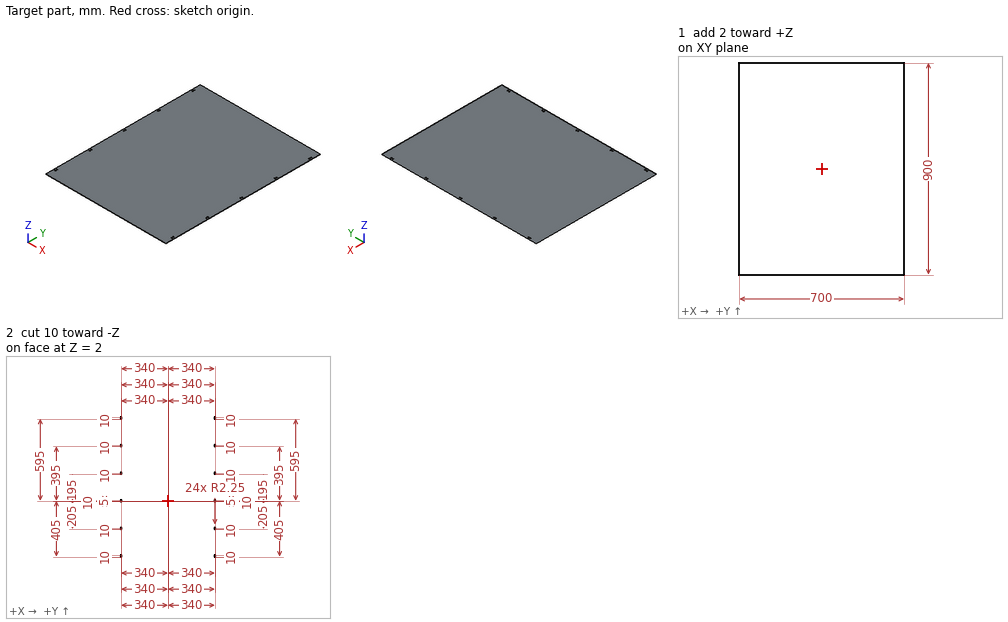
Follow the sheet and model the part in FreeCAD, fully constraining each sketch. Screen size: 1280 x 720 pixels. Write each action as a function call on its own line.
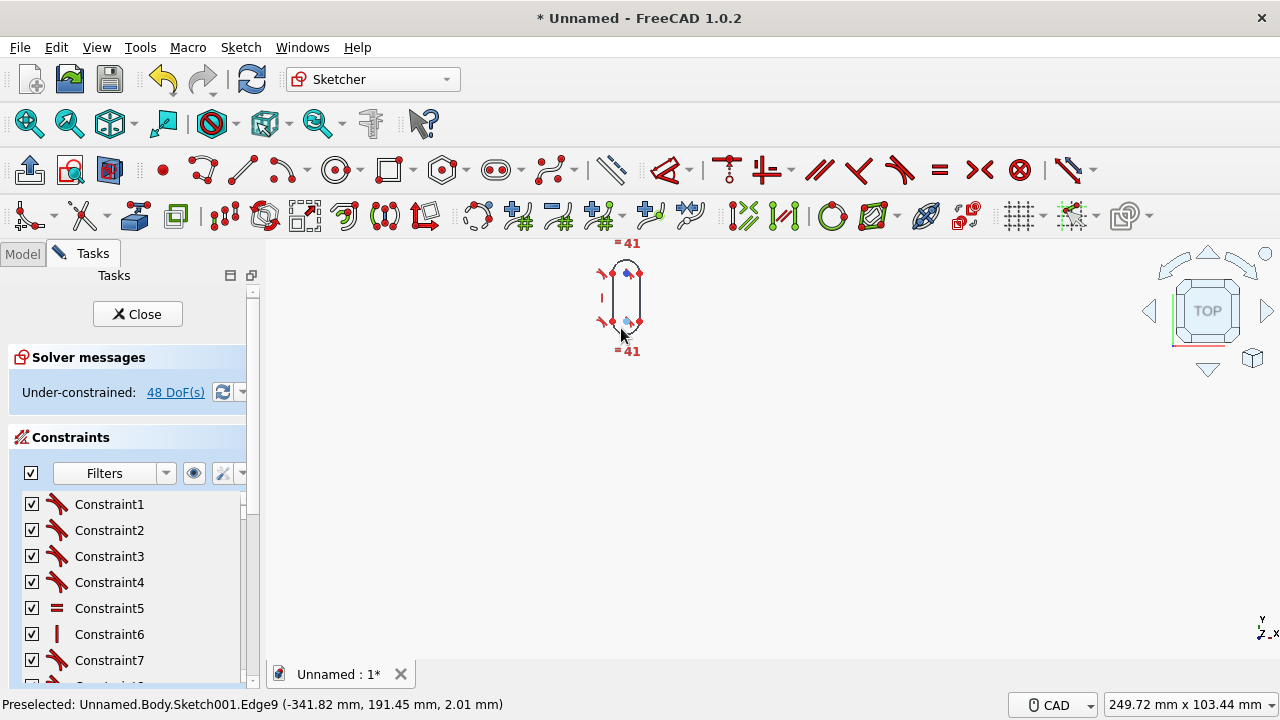
click(618, 332)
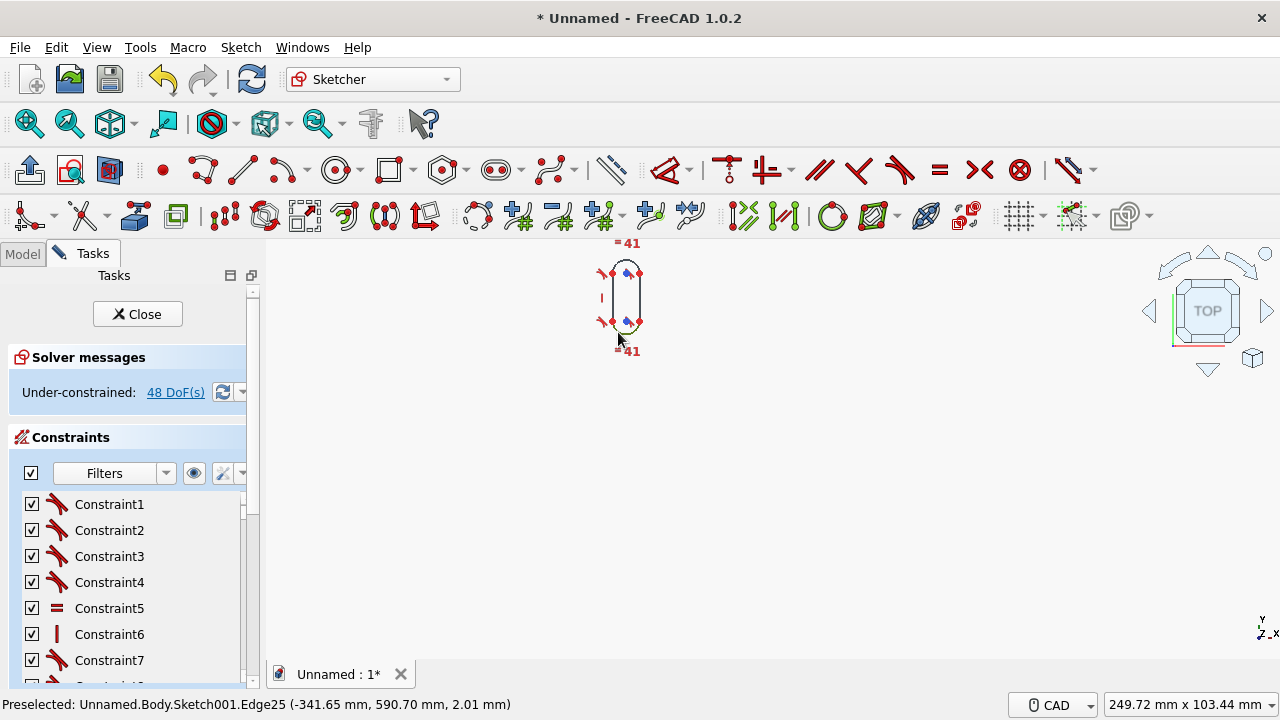
scroll(620, 328, down, 14)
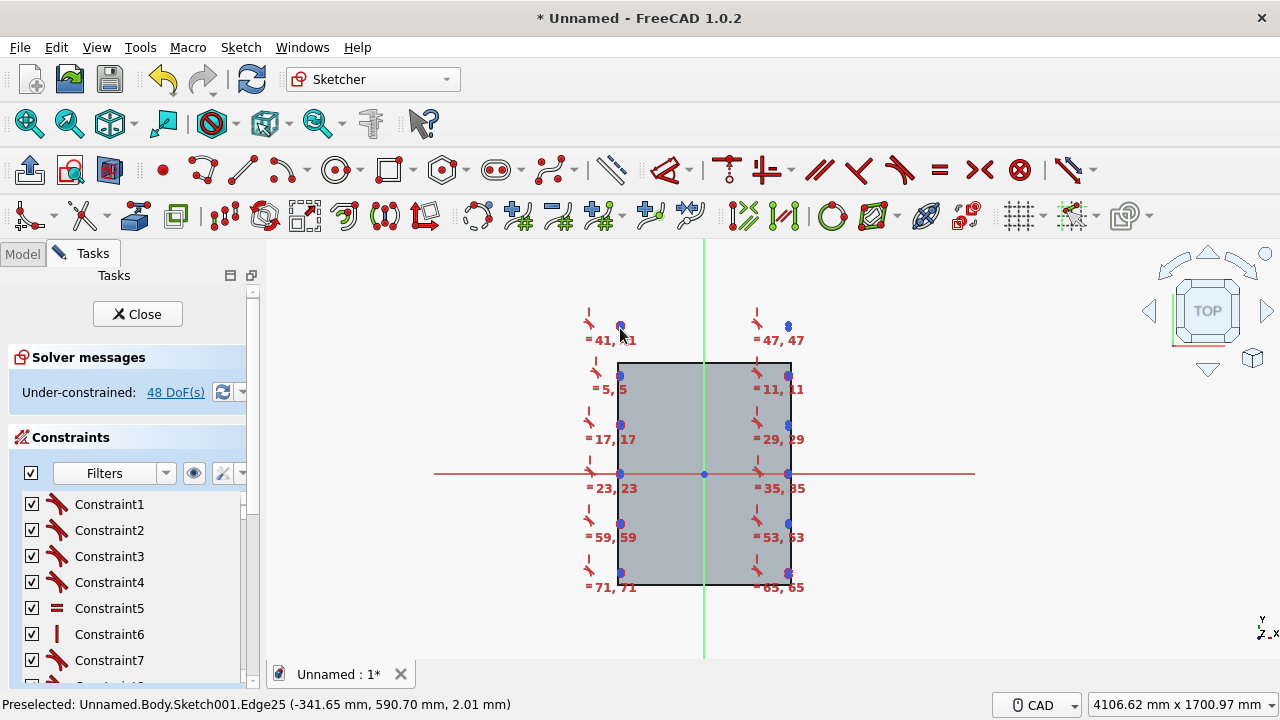
scroll(789, 328, up, 14)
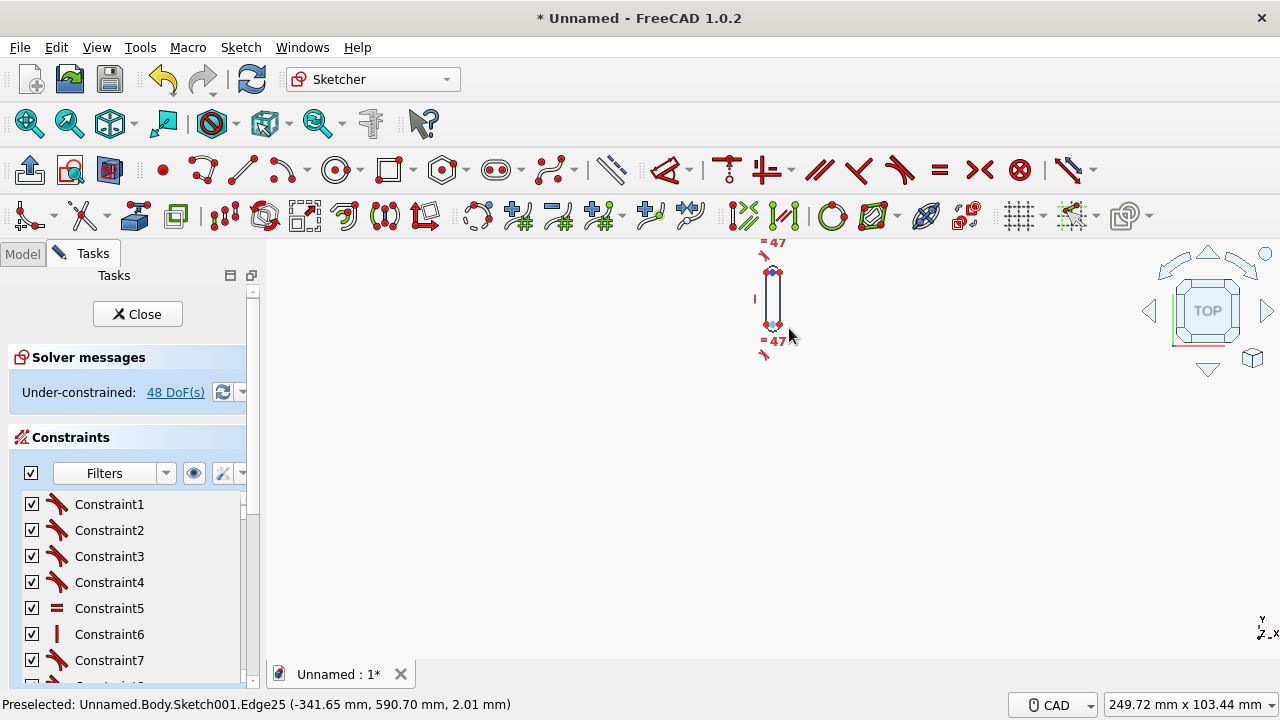
click(773, 332)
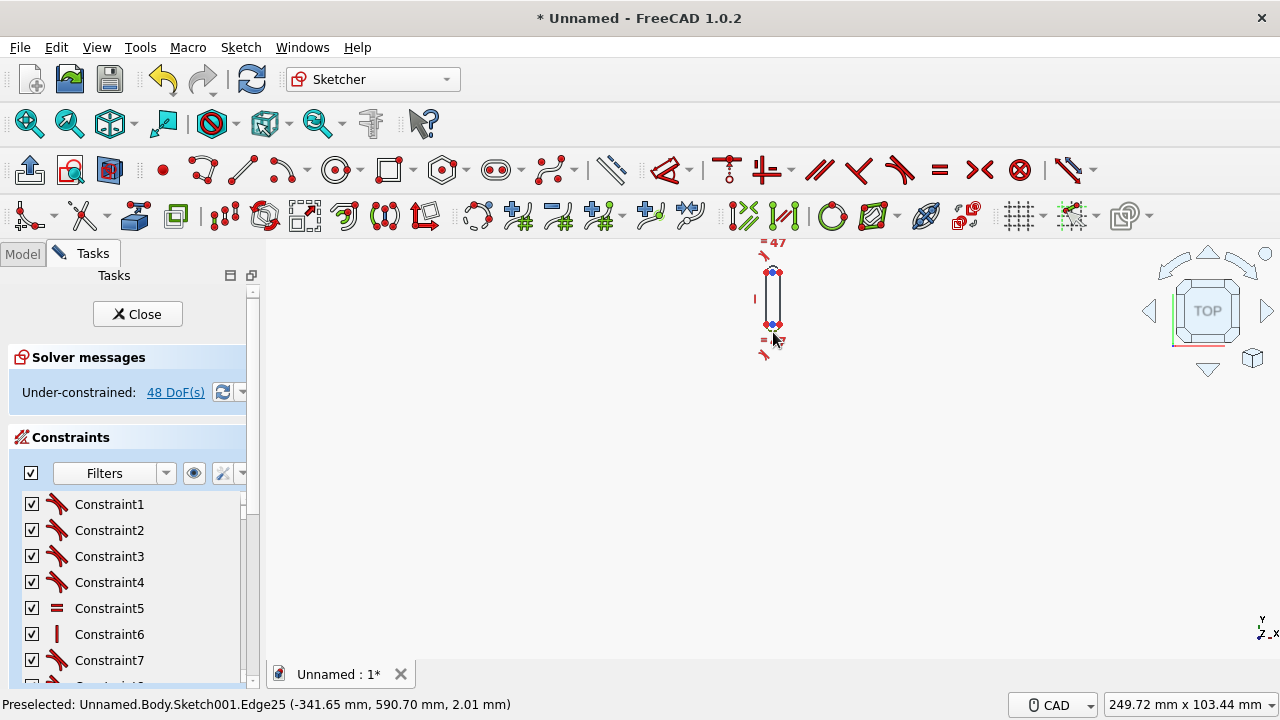
scroll(790, 328, down, 14)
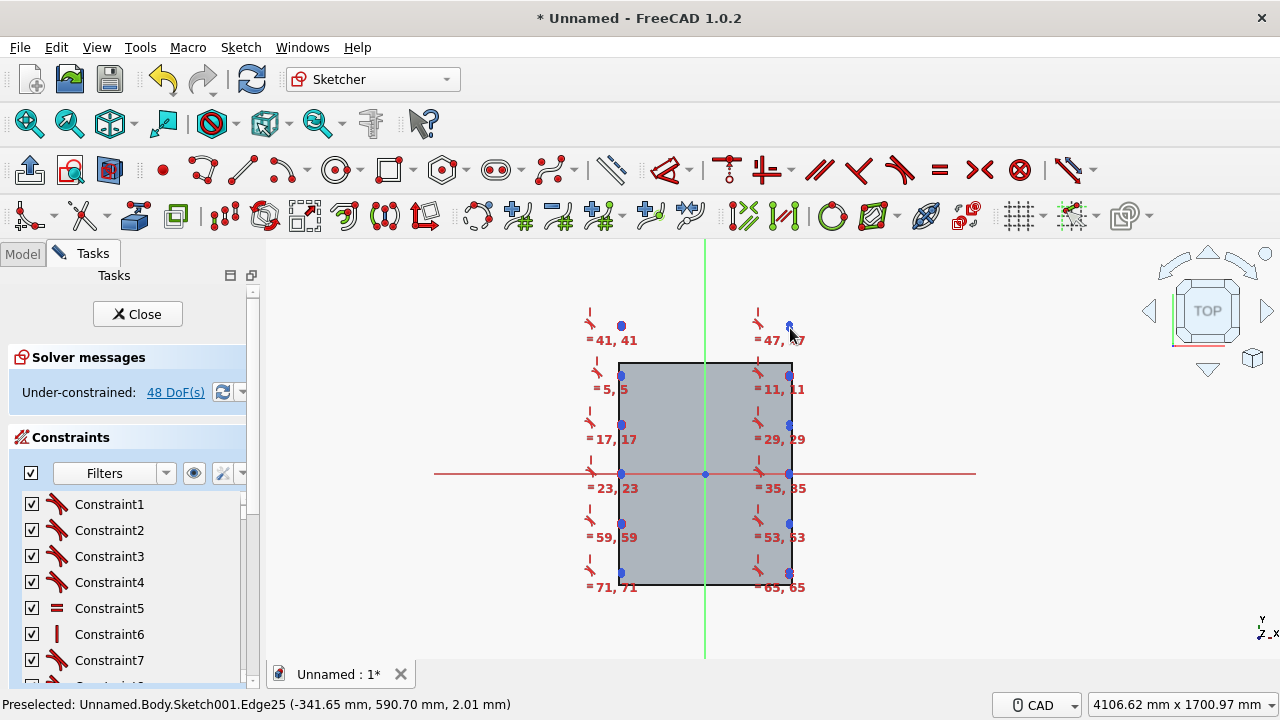
scroll(789, 526, up, 14)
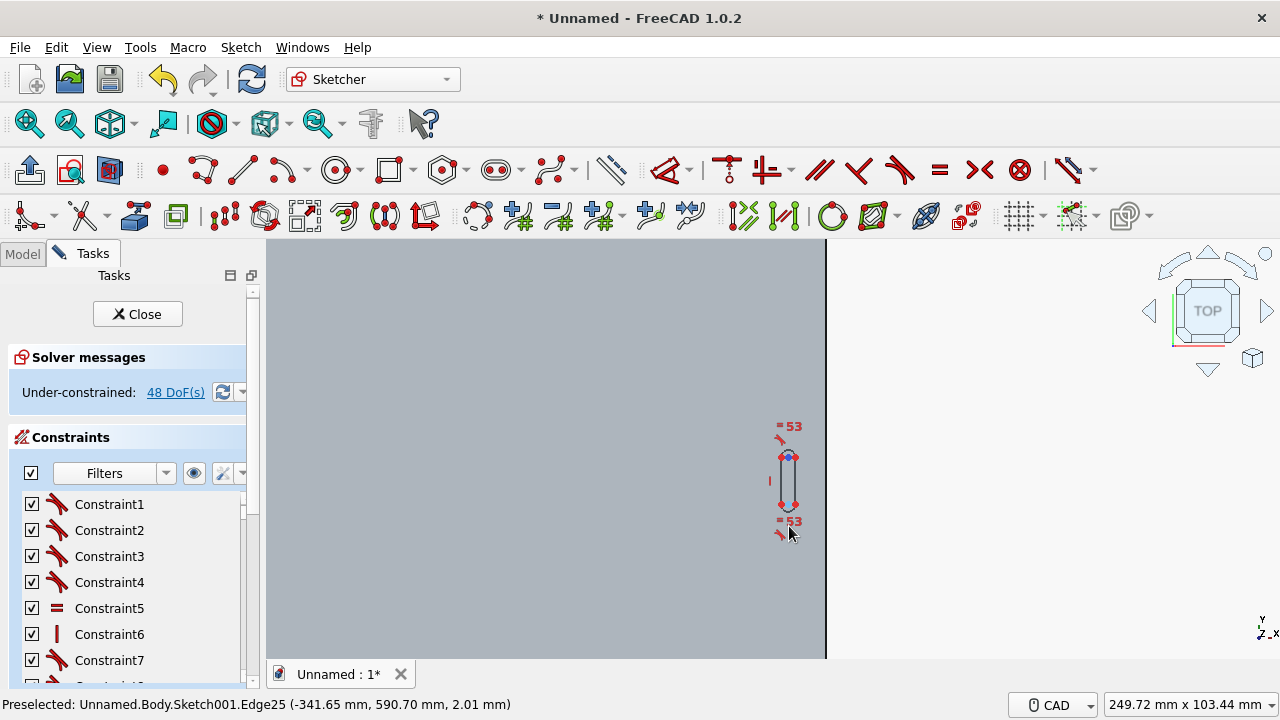
click(788, 512)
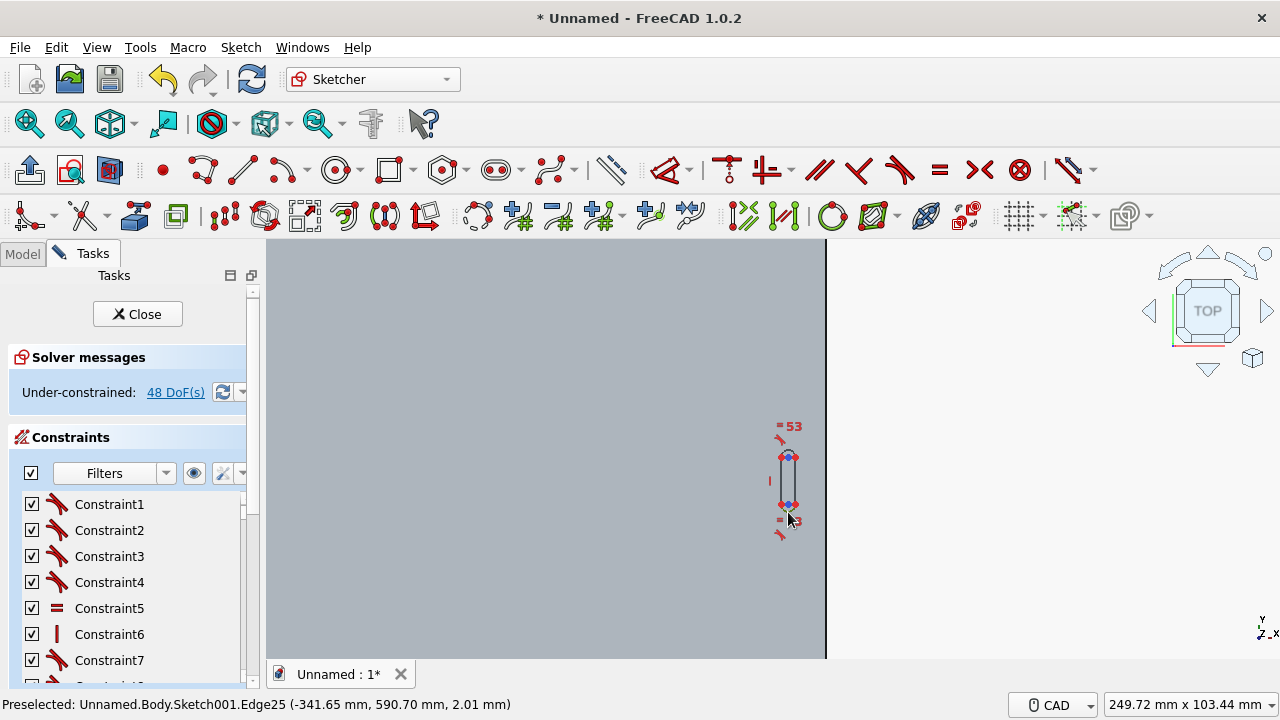
scroll(789, 526, down, 14)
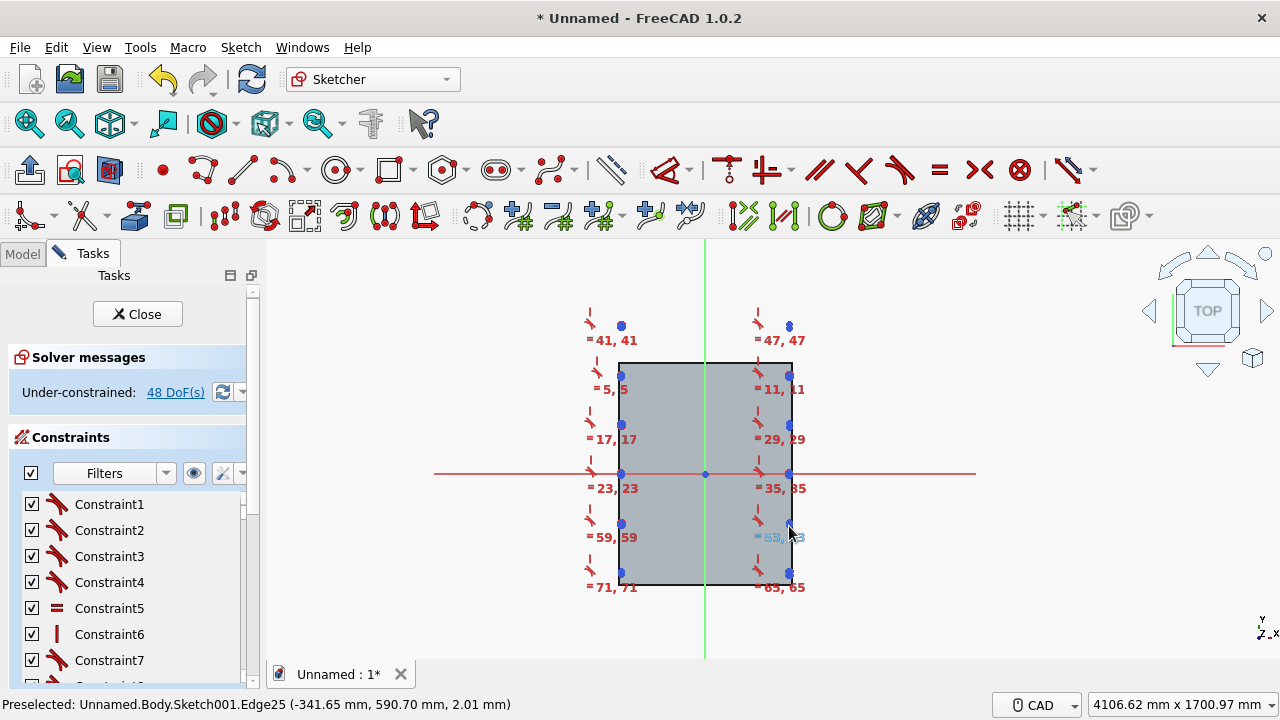
scroll(621, 526, up, 14)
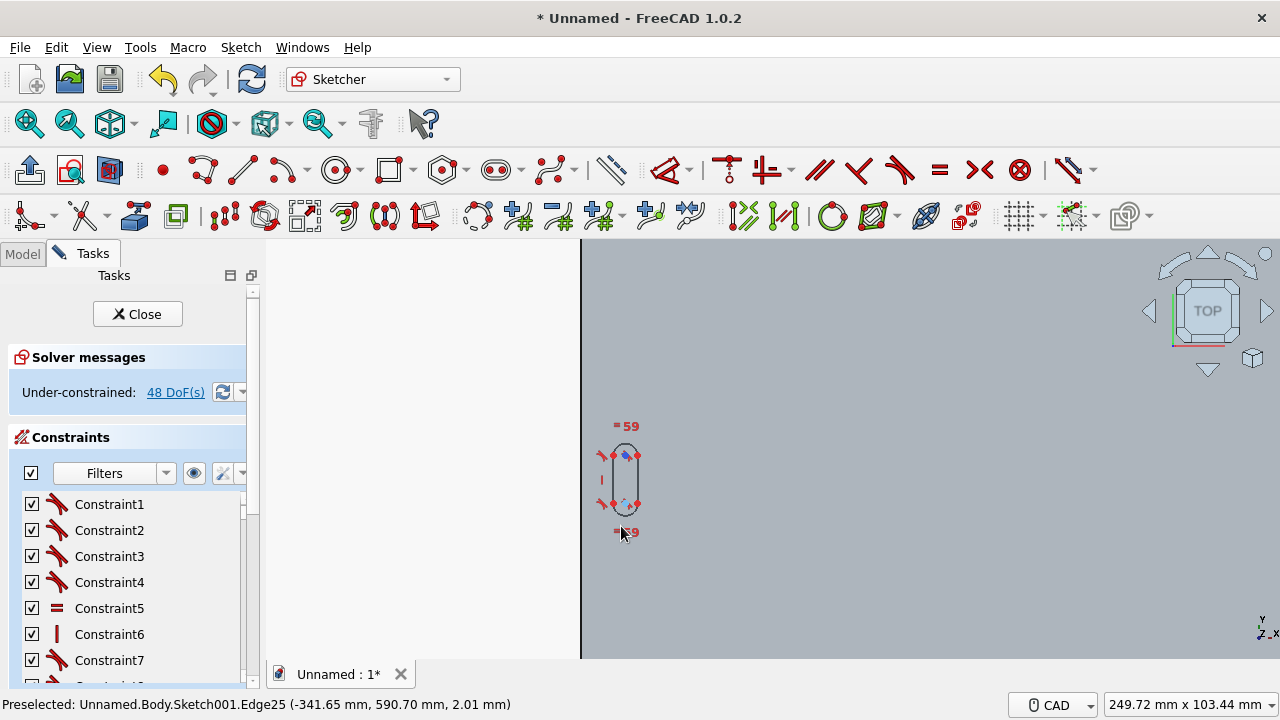
click(618, 514)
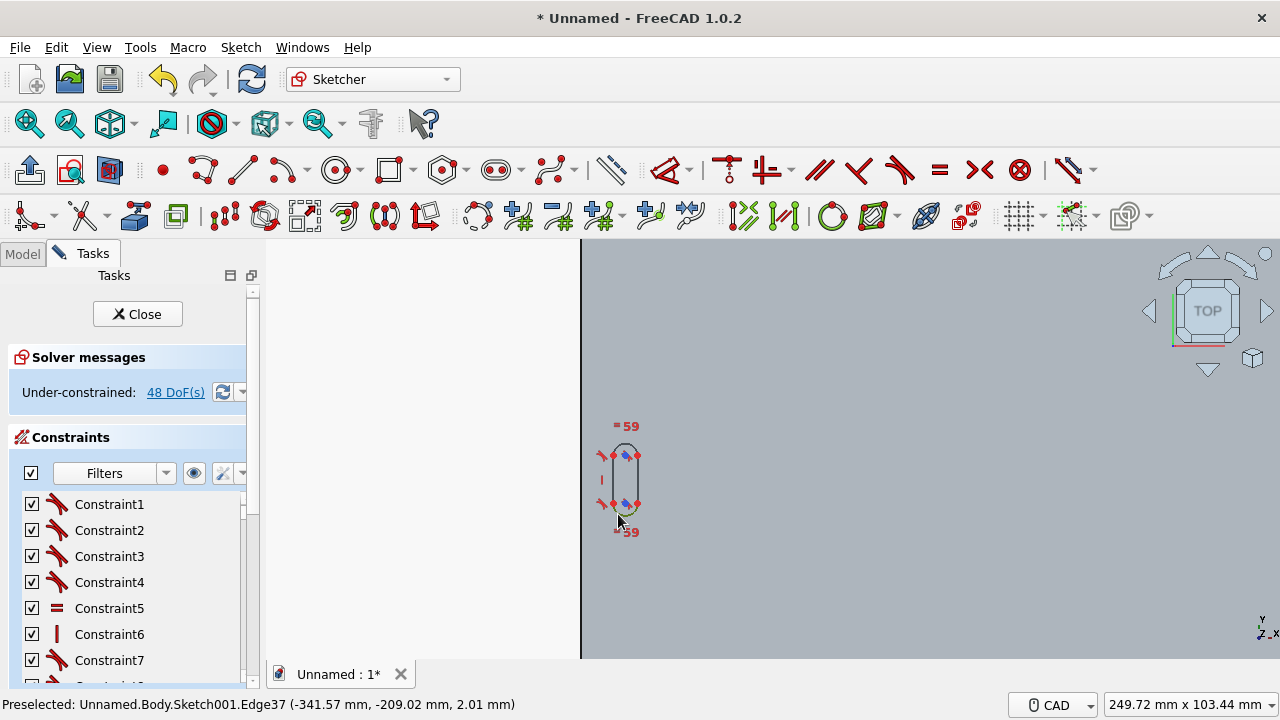
scroll(620, 526, down, 14)